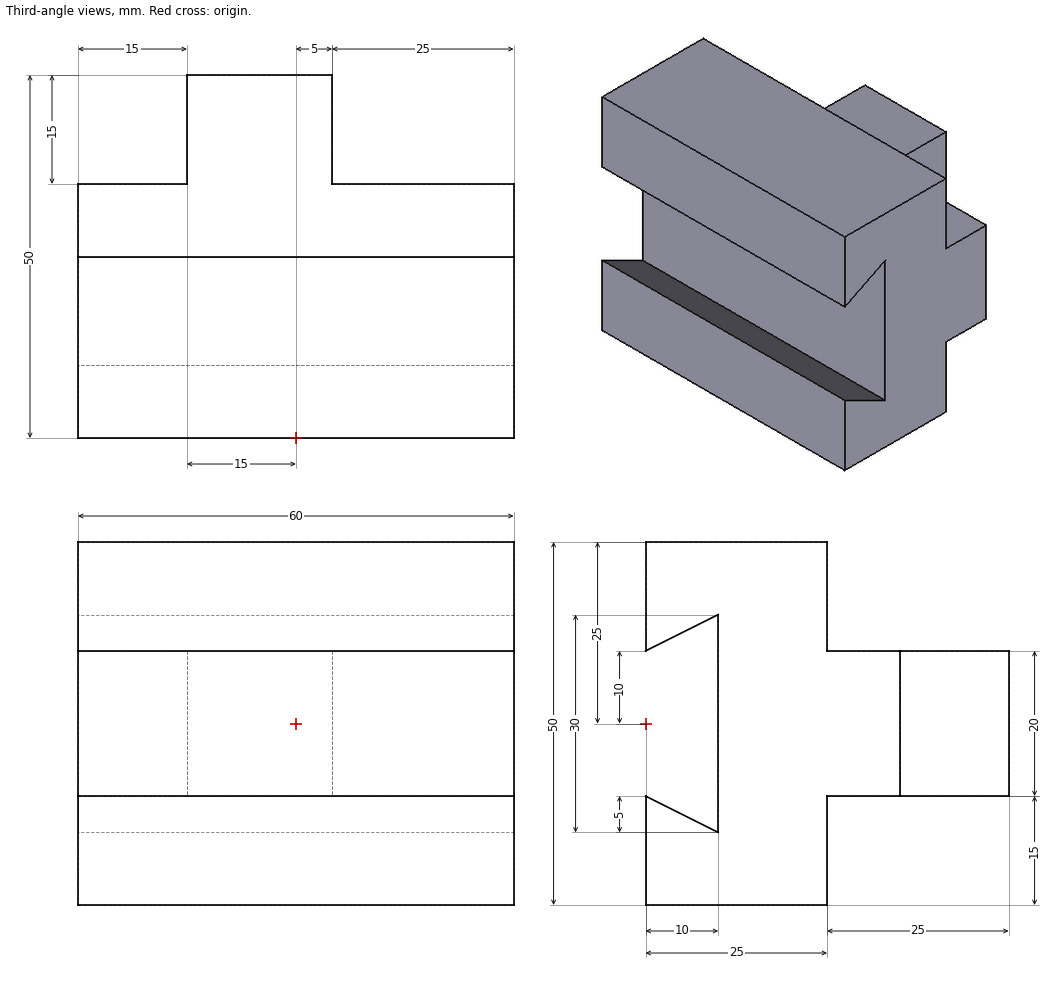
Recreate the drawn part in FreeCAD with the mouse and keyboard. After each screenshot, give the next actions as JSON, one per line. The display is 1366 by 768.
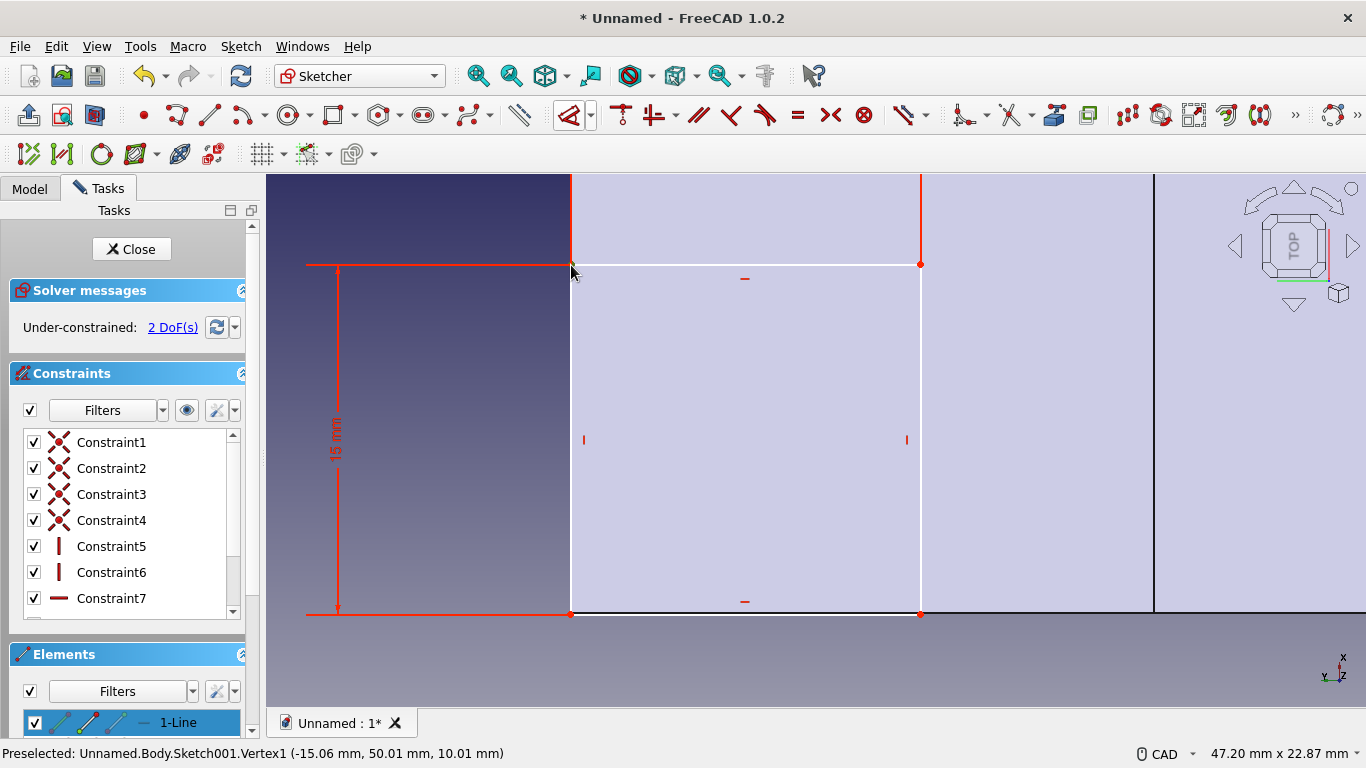
{"action": "key", "text": "l"}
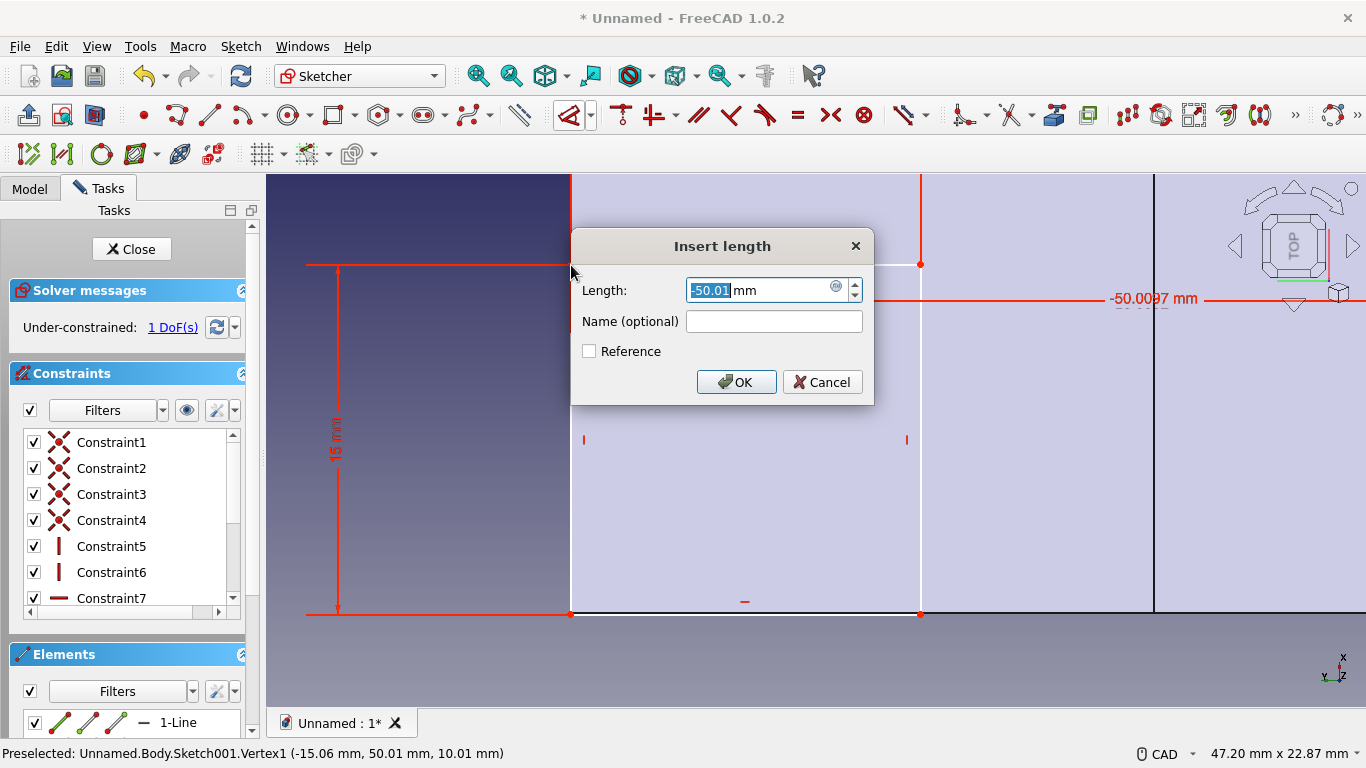
{"action": "type", "text": "-50"}
{"action": "key", "text": "Return"}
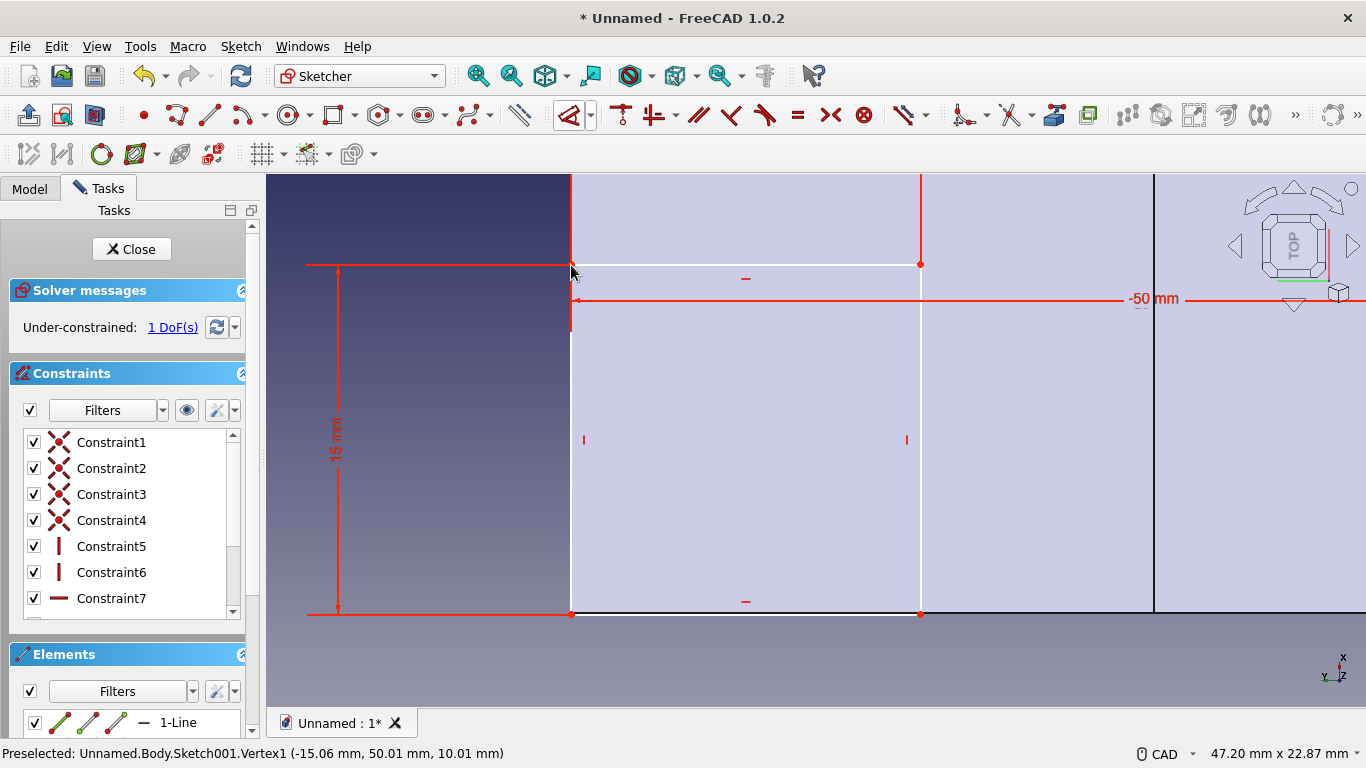
{"action": "left_click", "coordinate": [571, 265]}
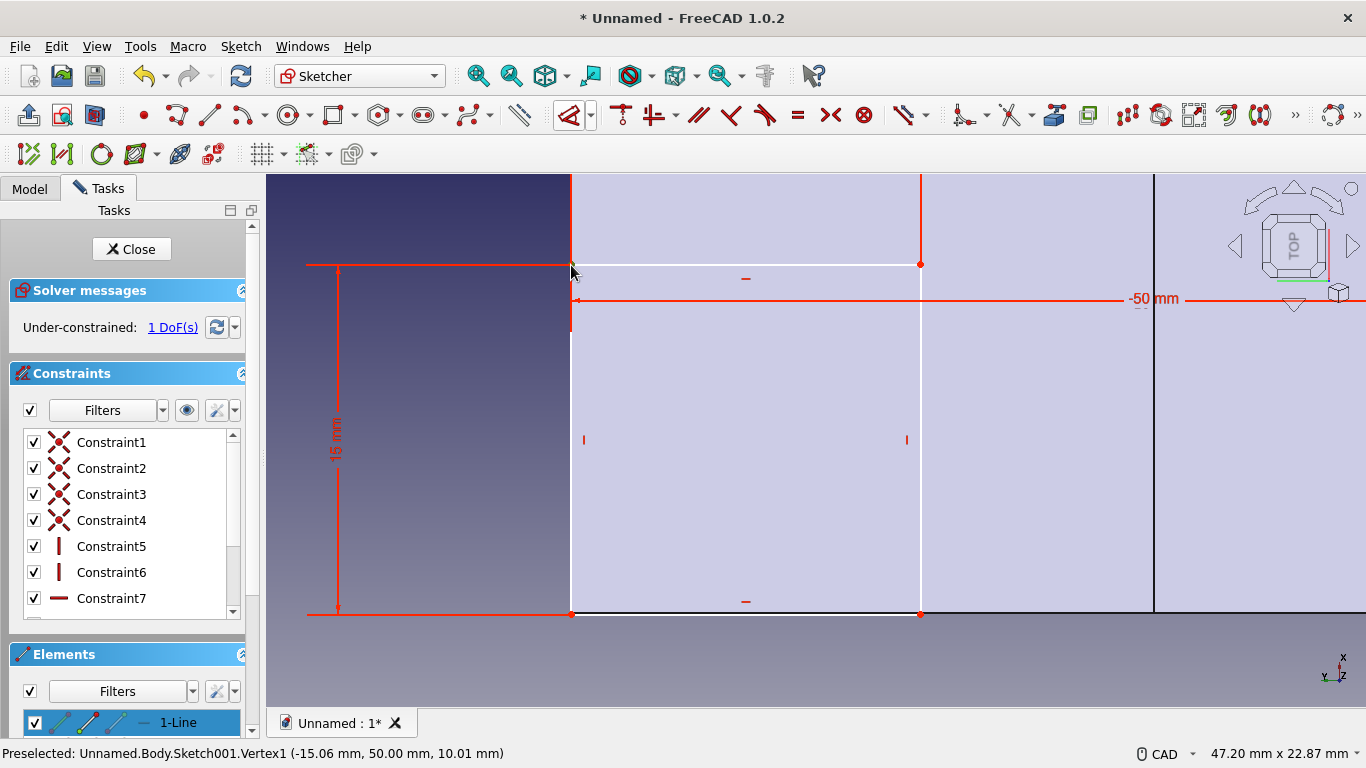
{"action": "key", "text": "i"}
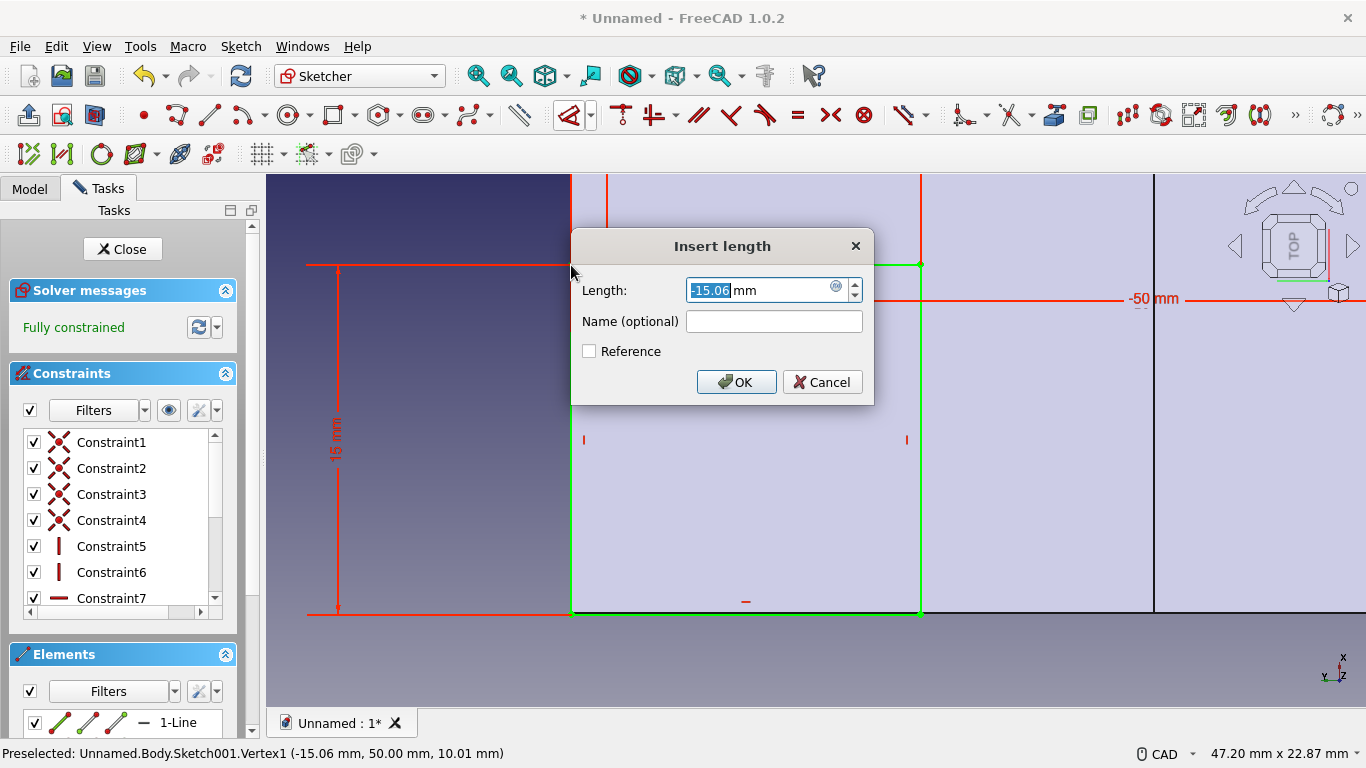
{"action": "type", "text": "-15"}
{"action": "key", "text": "Return"}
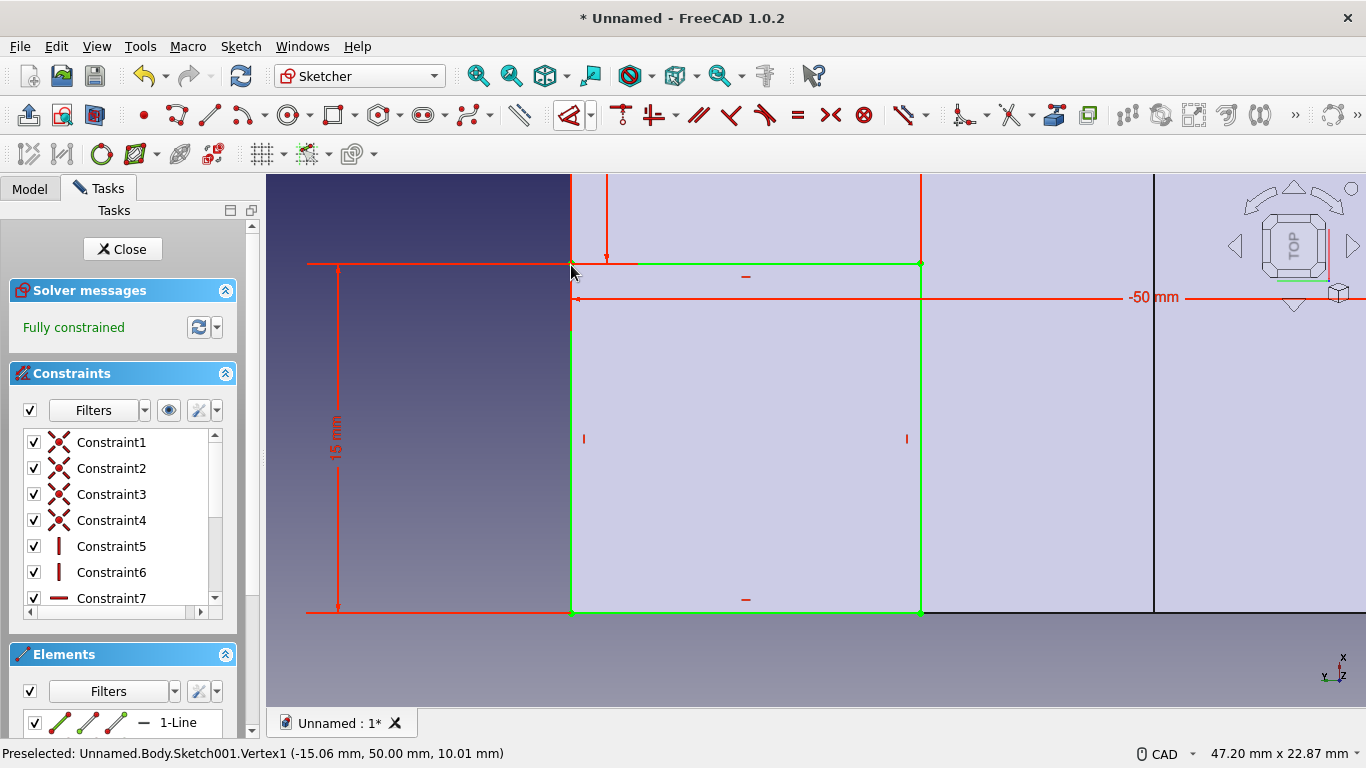
{"action": "left_click", "coordinate": [123, 249]}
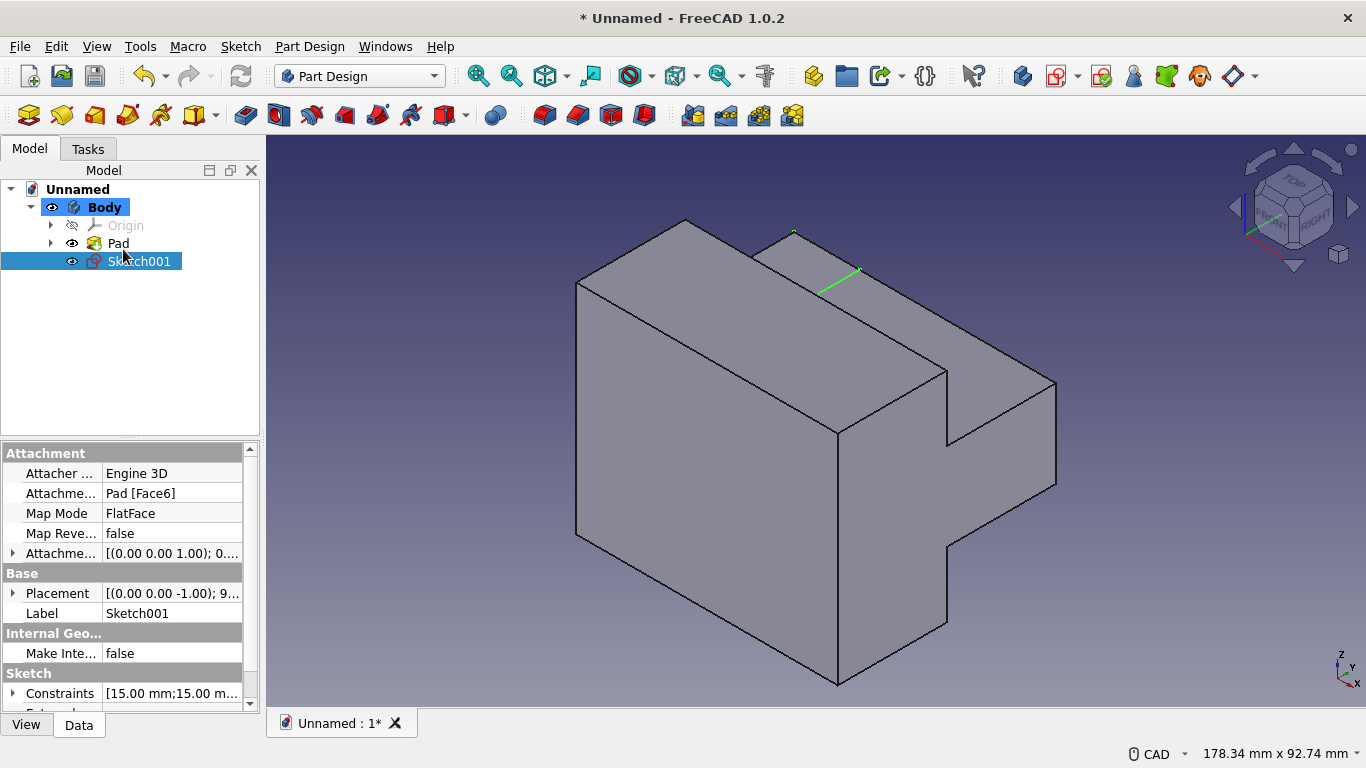
{"action": "left_click", "coordinate": [246, 116]}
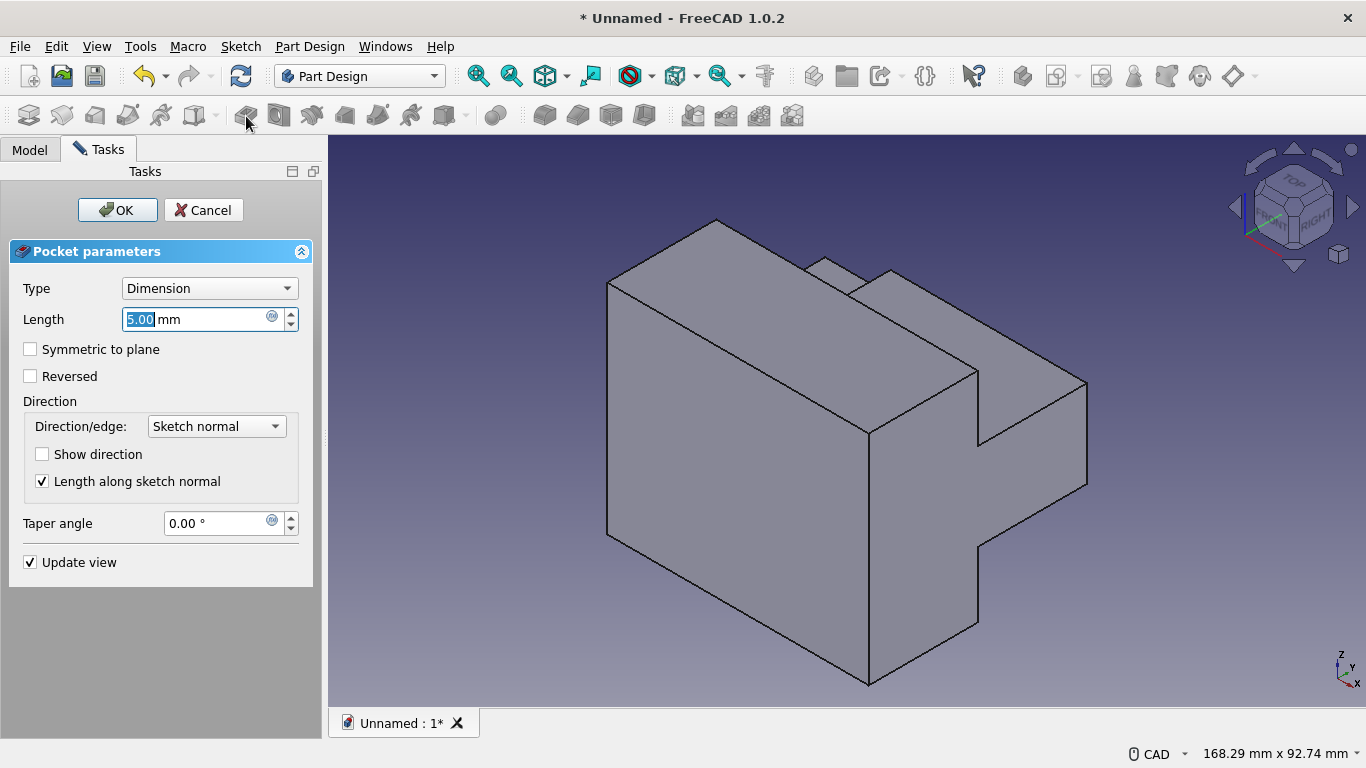
{"action": "left_click", "coordinate": [210, 288]}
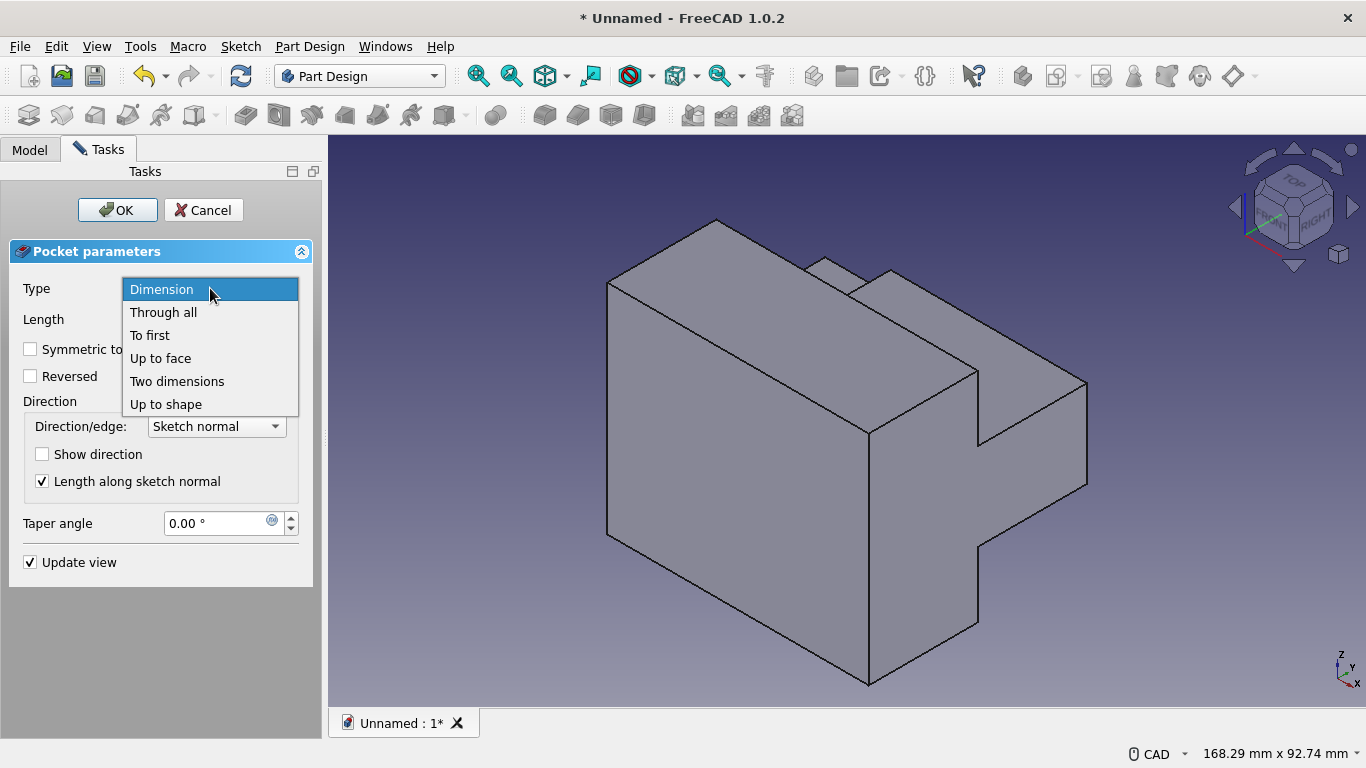
{"action": "left_click", "coordinate": [208, 336]}